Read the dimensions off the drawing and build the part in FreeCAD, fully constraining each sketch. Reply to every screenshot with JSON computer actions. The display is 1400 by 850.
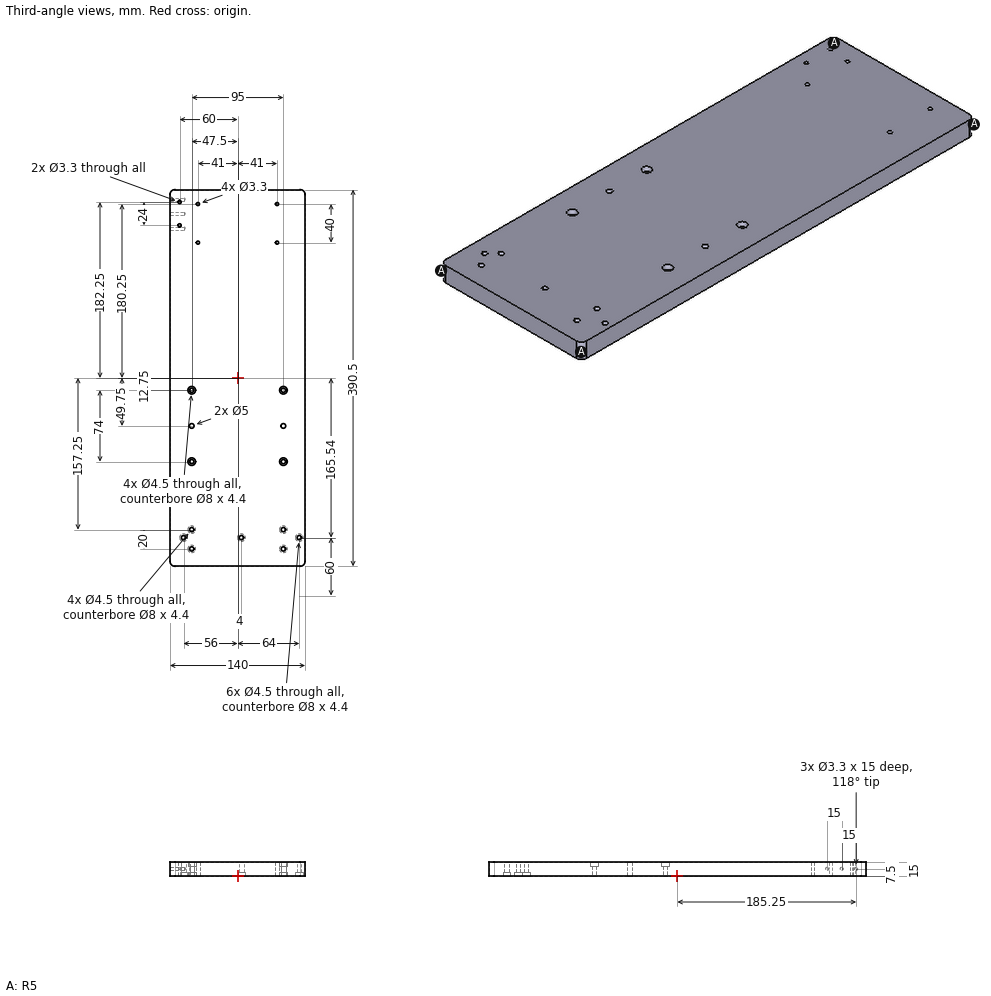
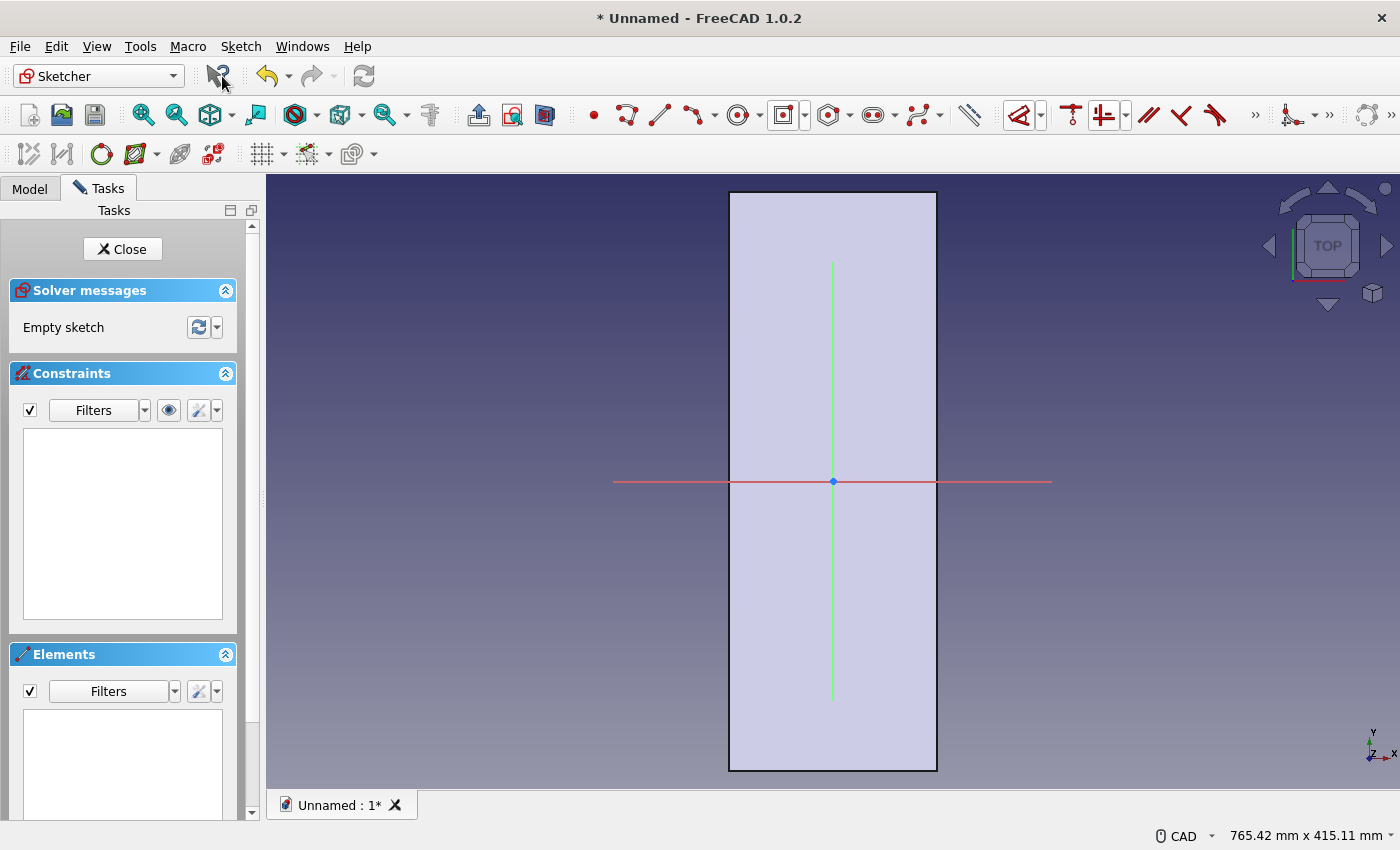
{"action": "scroll", "coordinate": [873, 586], "scroll_direction": "up", "scroll_amount": 5}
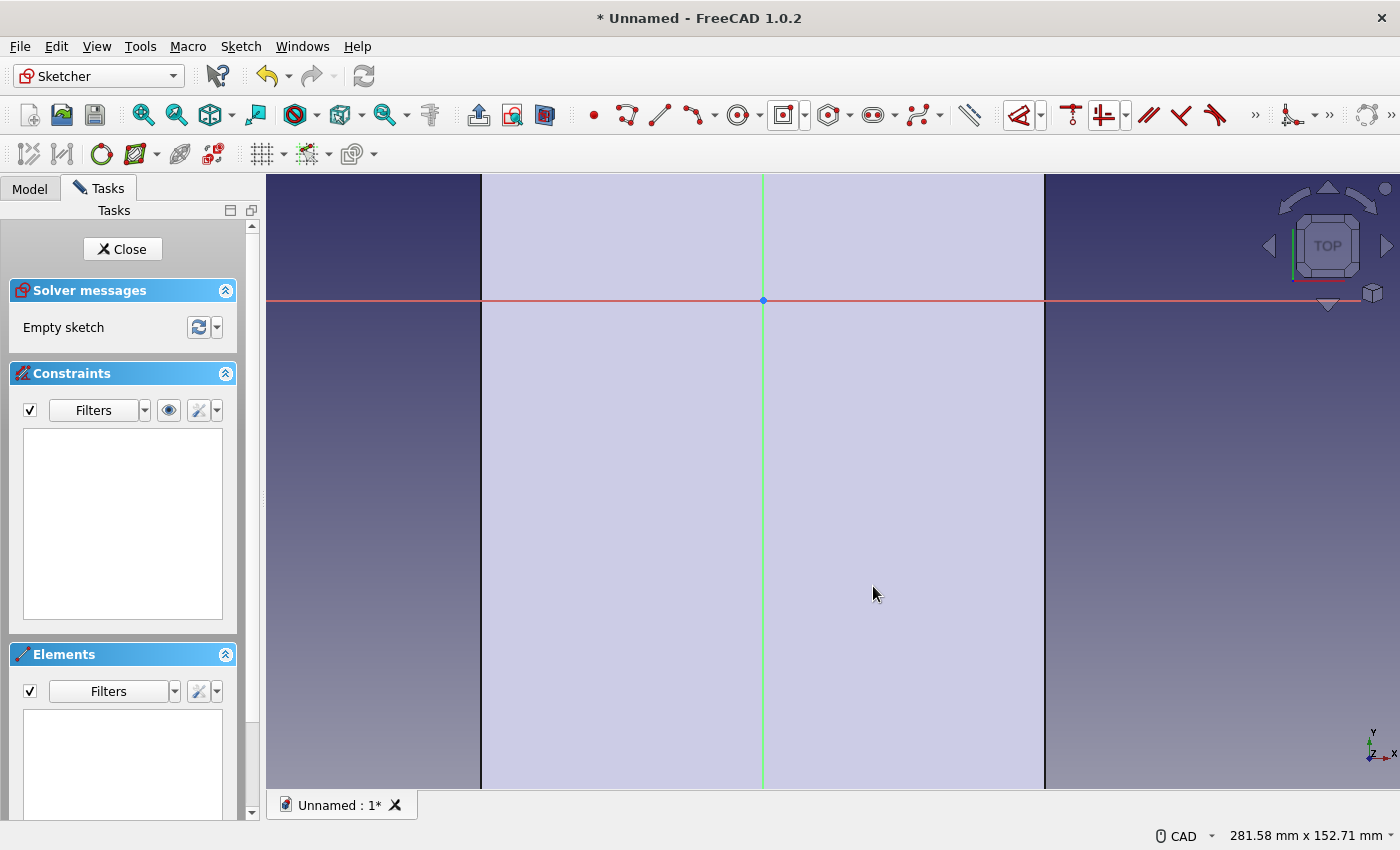
{"action": "left_click", "coordinate": [738, 116]}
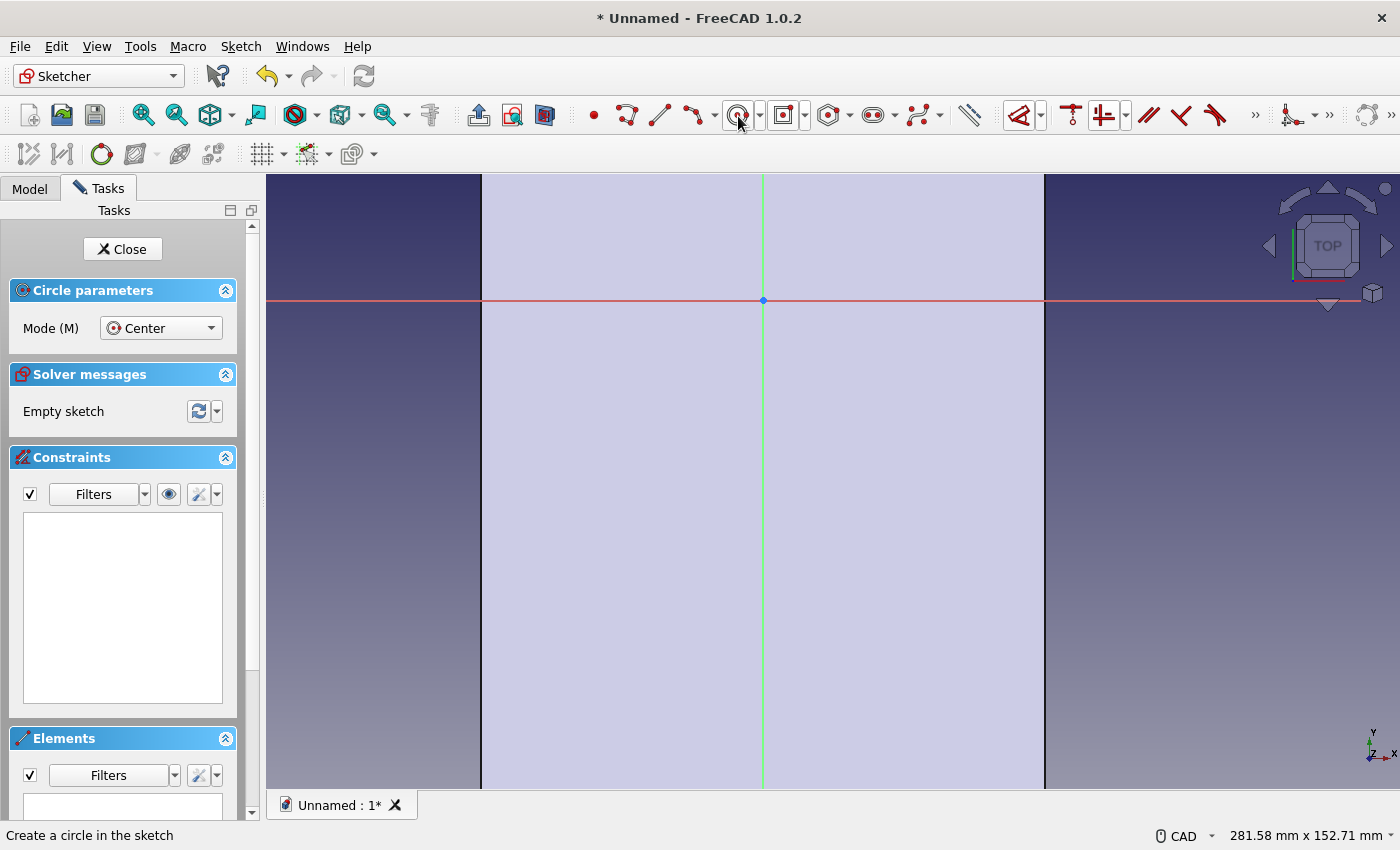
{"action": "scroll", "coordinate": [572, 352], "scroll_direction": "up", "scroll_amount": 5}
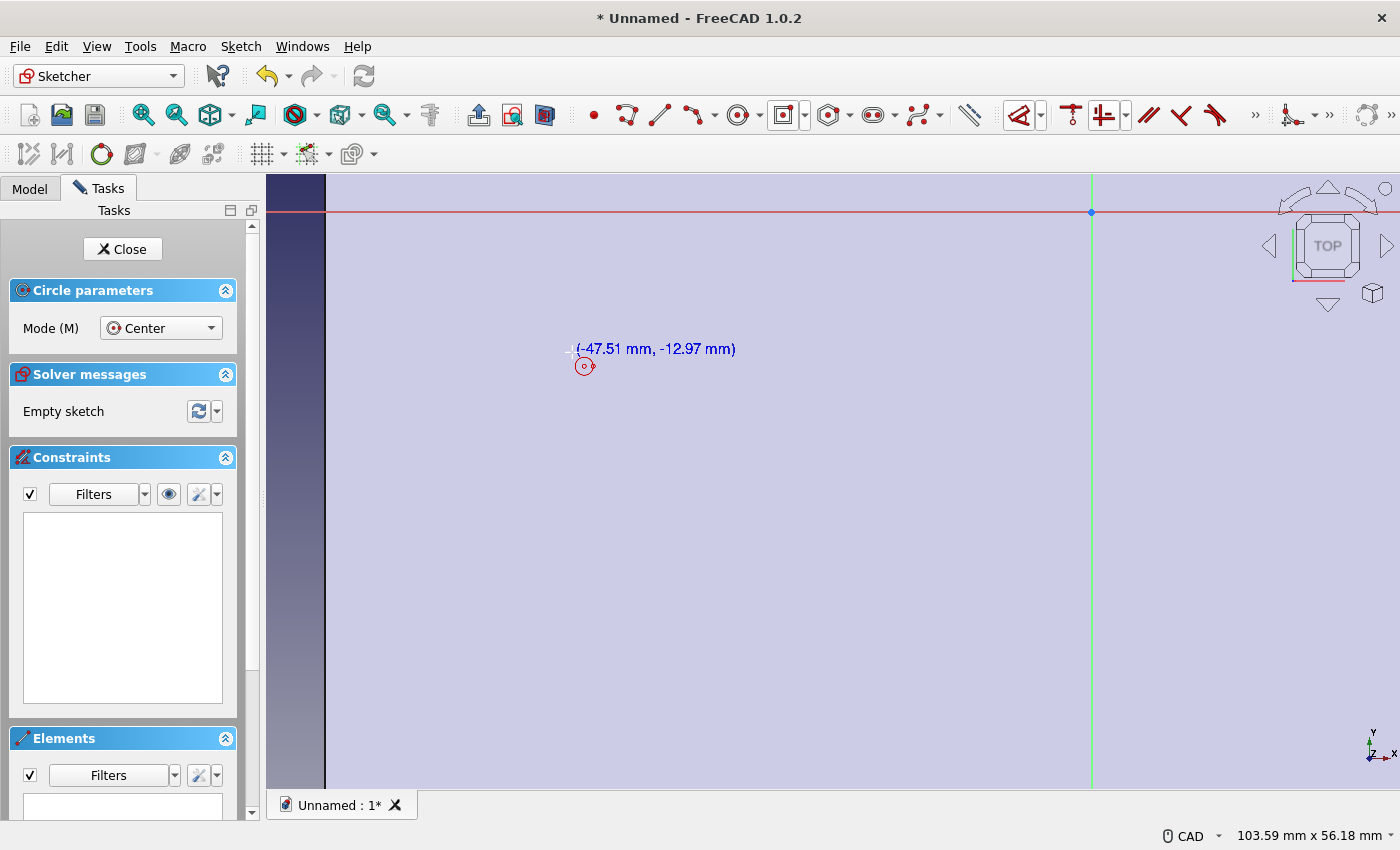
{"action": "left_click", "coordinate": [572, 352]}
{"action": "mouse_move", "coordinate": [589, 334]}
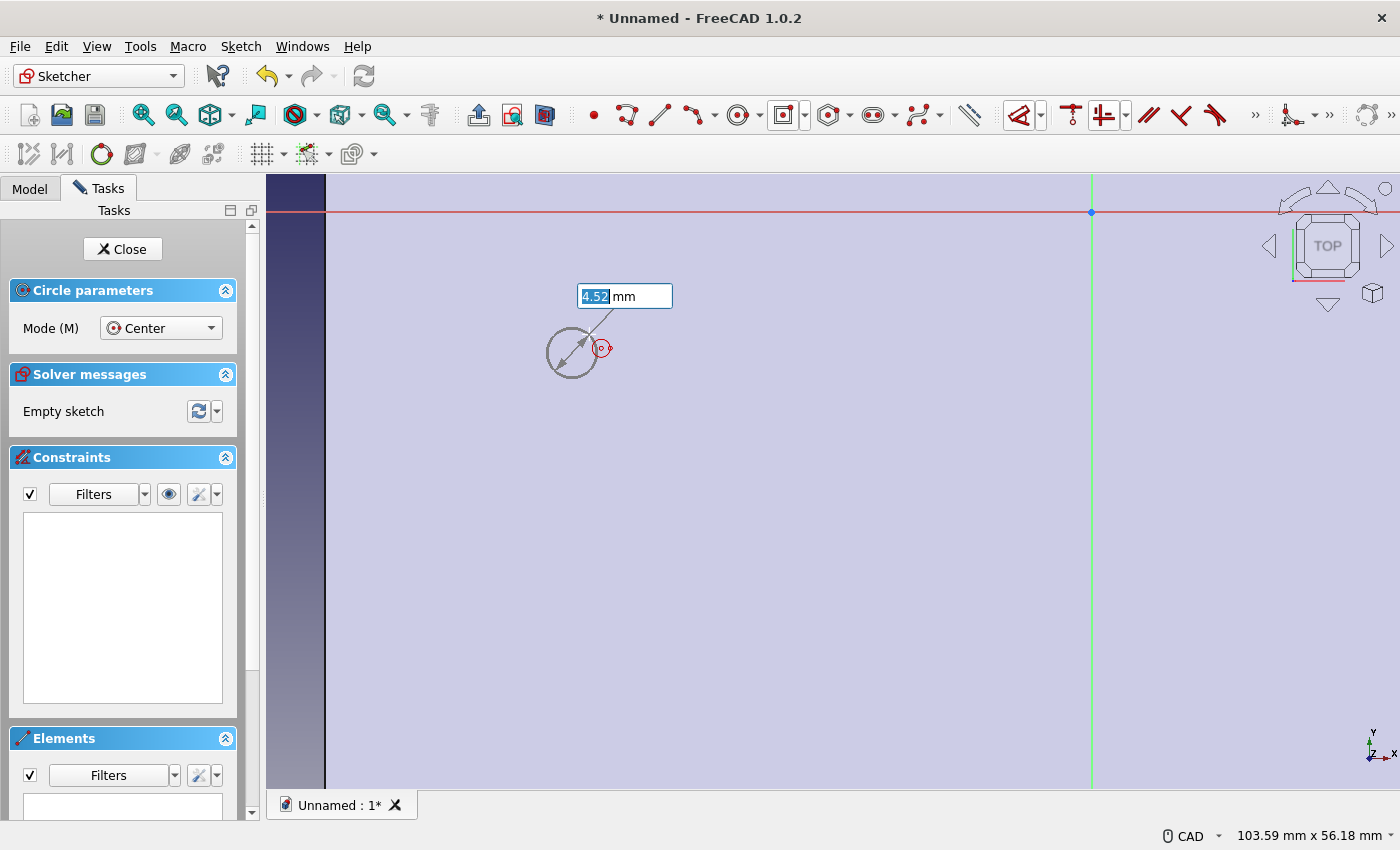
{"action": "type", "text": "4.5"}
{"action": "key", "text": "Return"}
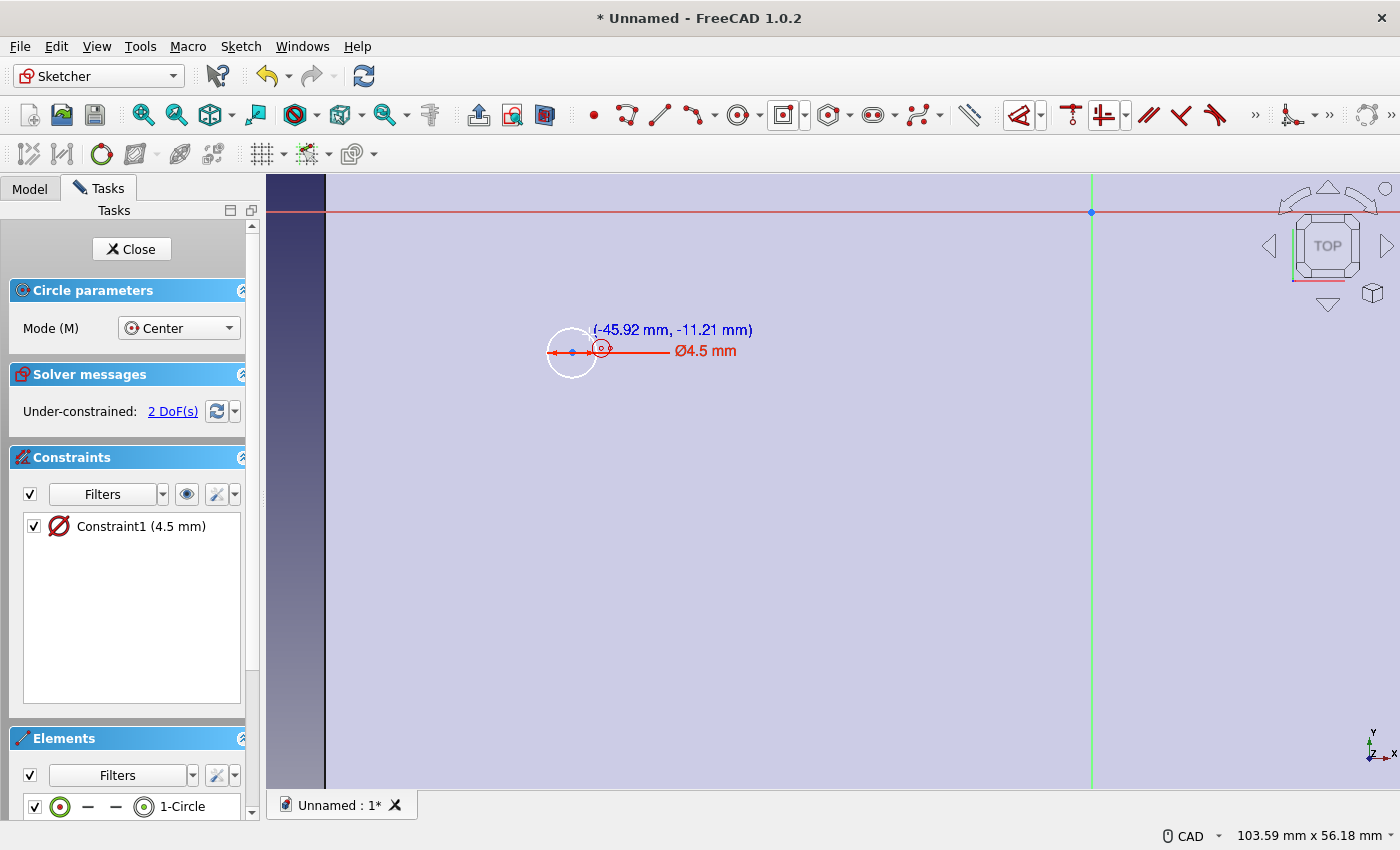
{"action": "scroll", "coordinate": [574, 355], "scroll_direction": "down", "scroll_amount": 5}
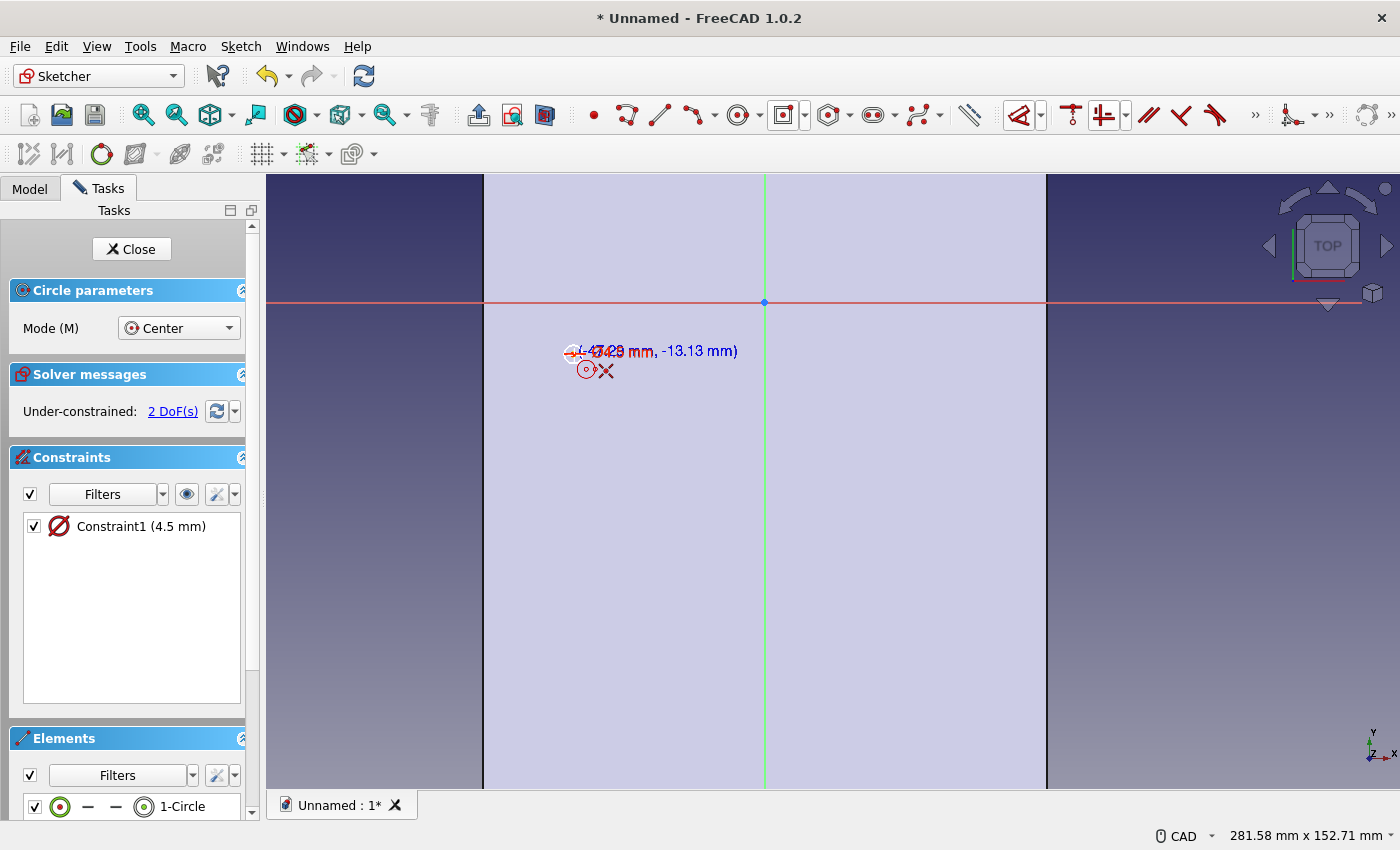
{"action": "scroll", "coordinate": [573, 652], "scroll_direction": "up", "scroll_amount": 5}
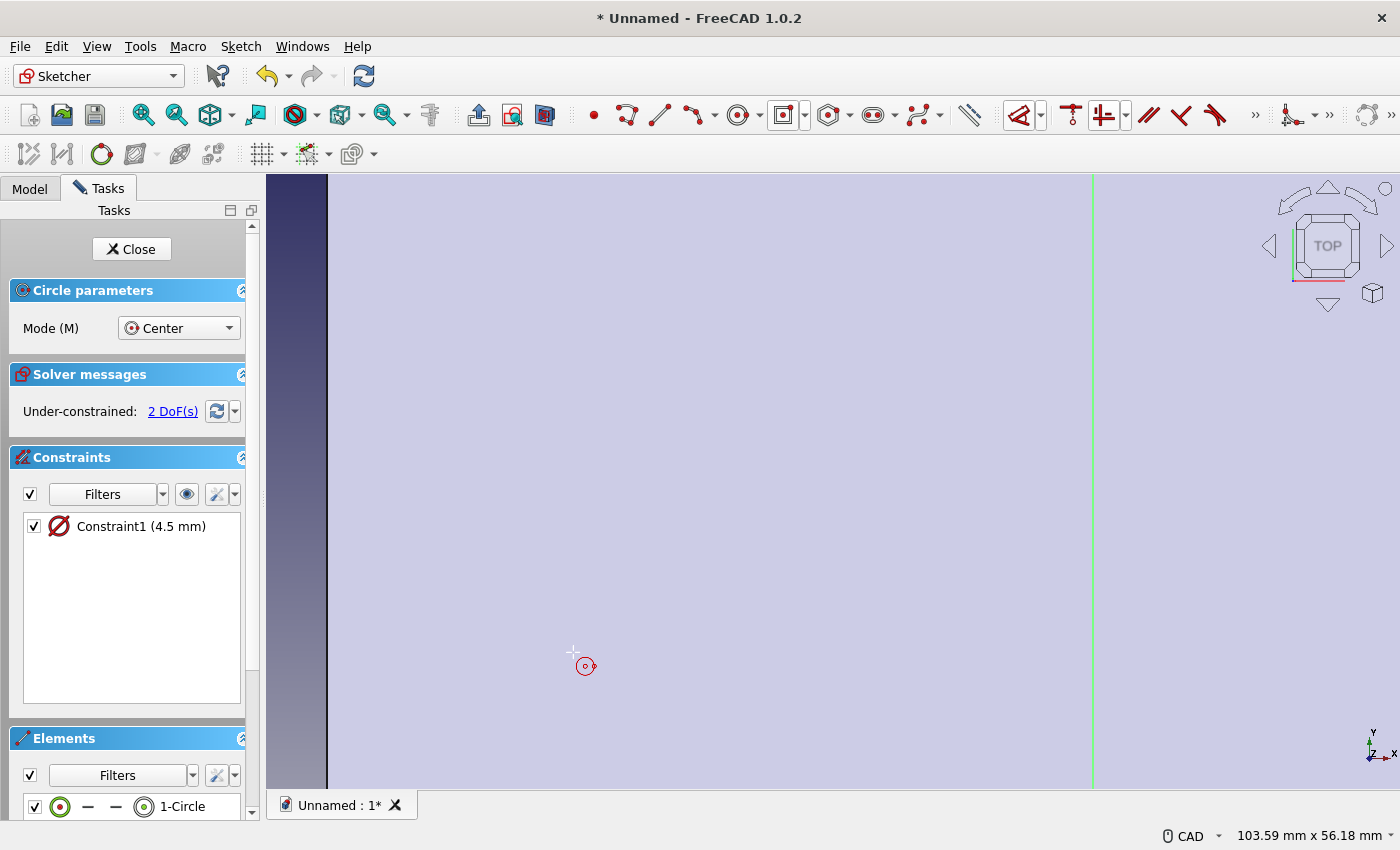
{"action": "left_click", "coordinate": [573, 651]}
{"action": "mouse_move", "coordinate": [591, 633]}